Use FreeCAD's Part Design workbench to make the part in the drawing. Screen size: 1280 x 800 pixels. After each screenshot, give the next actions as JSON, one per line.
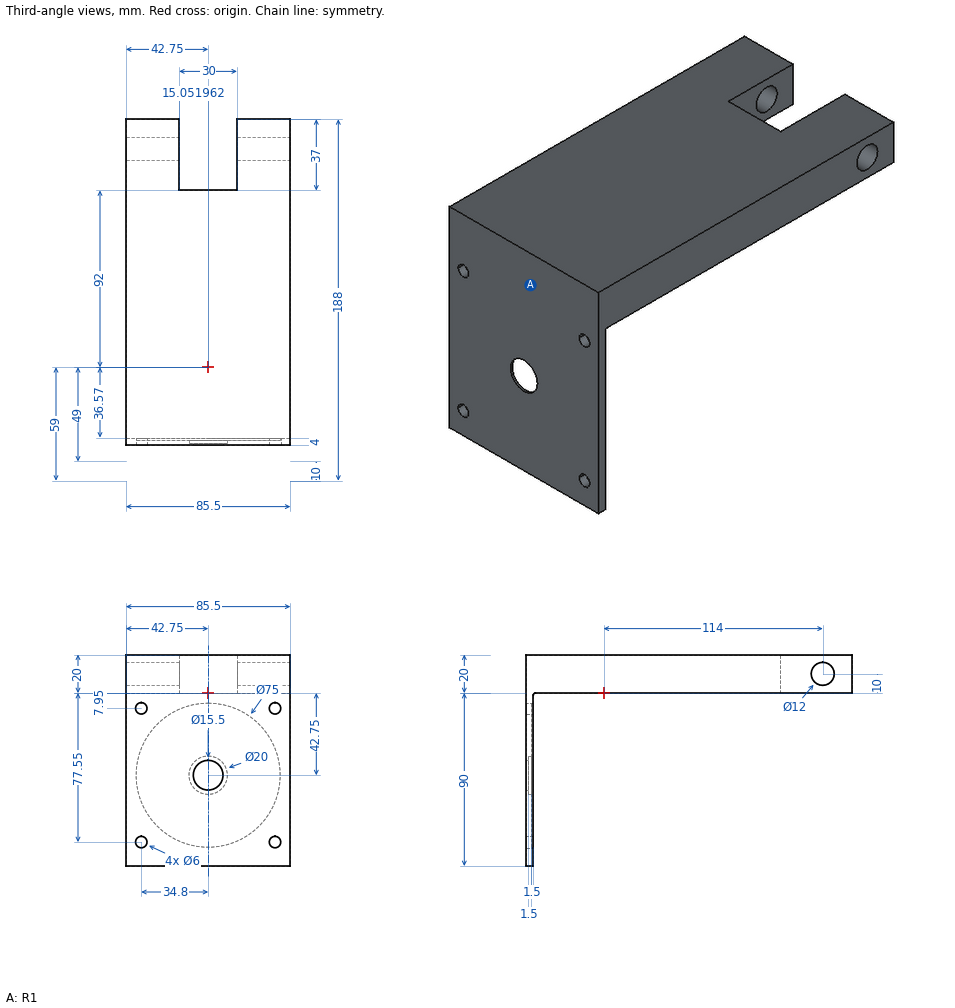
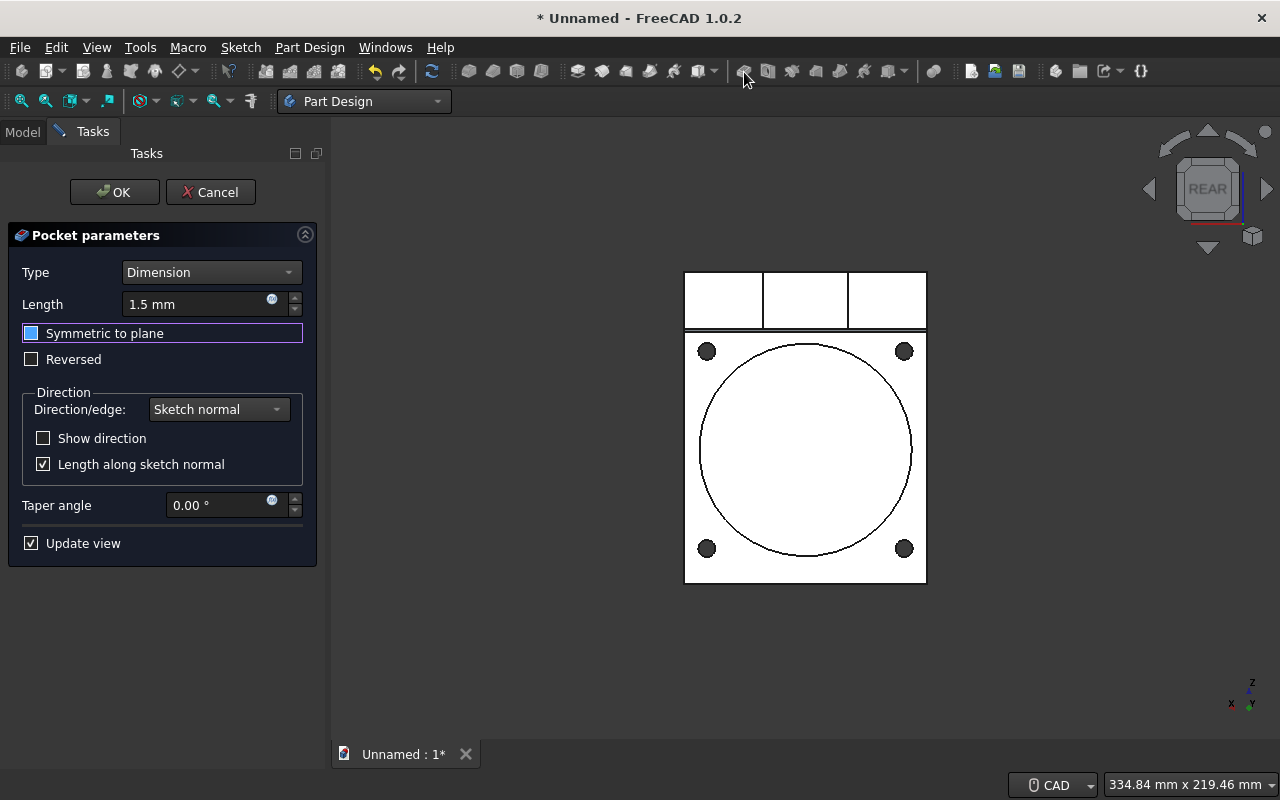
{"action": "left_click", "coordinate": [115, 192]}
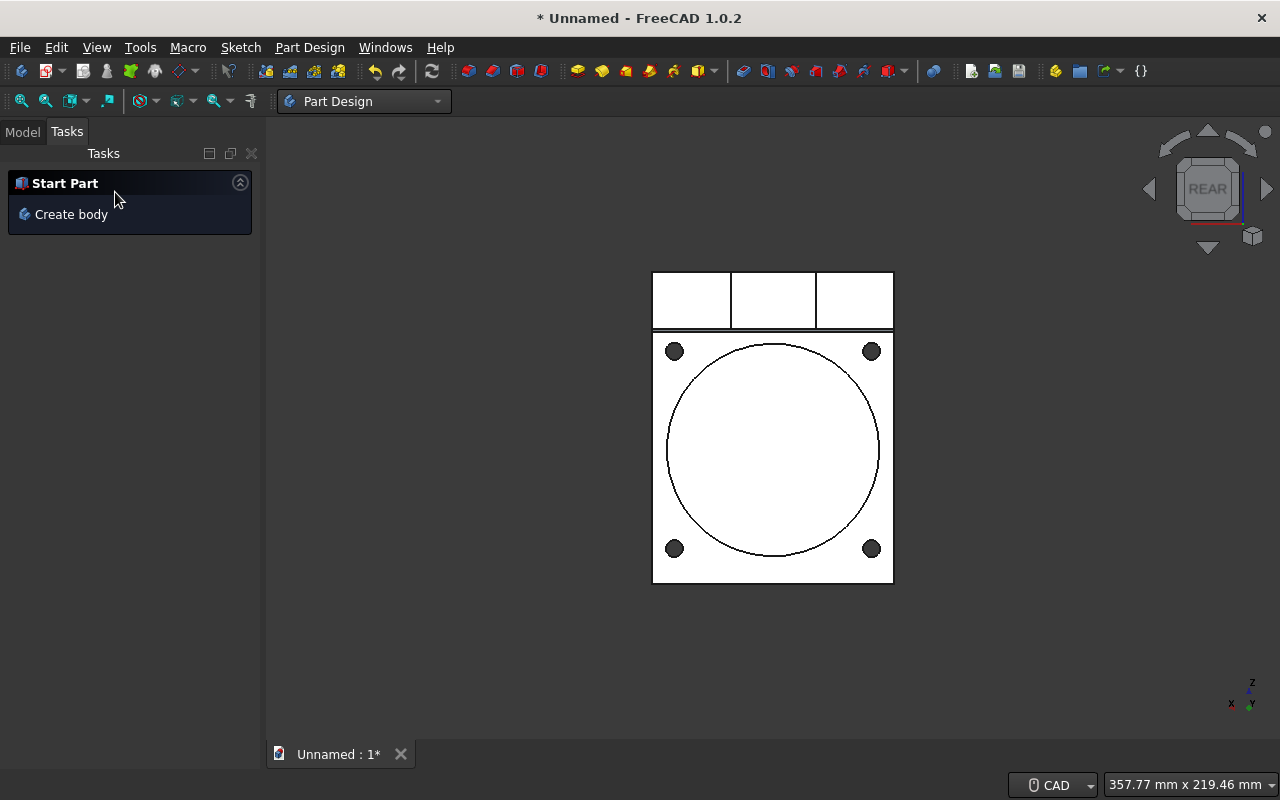
{"action": "left_click", "coordinate": [773, 449]}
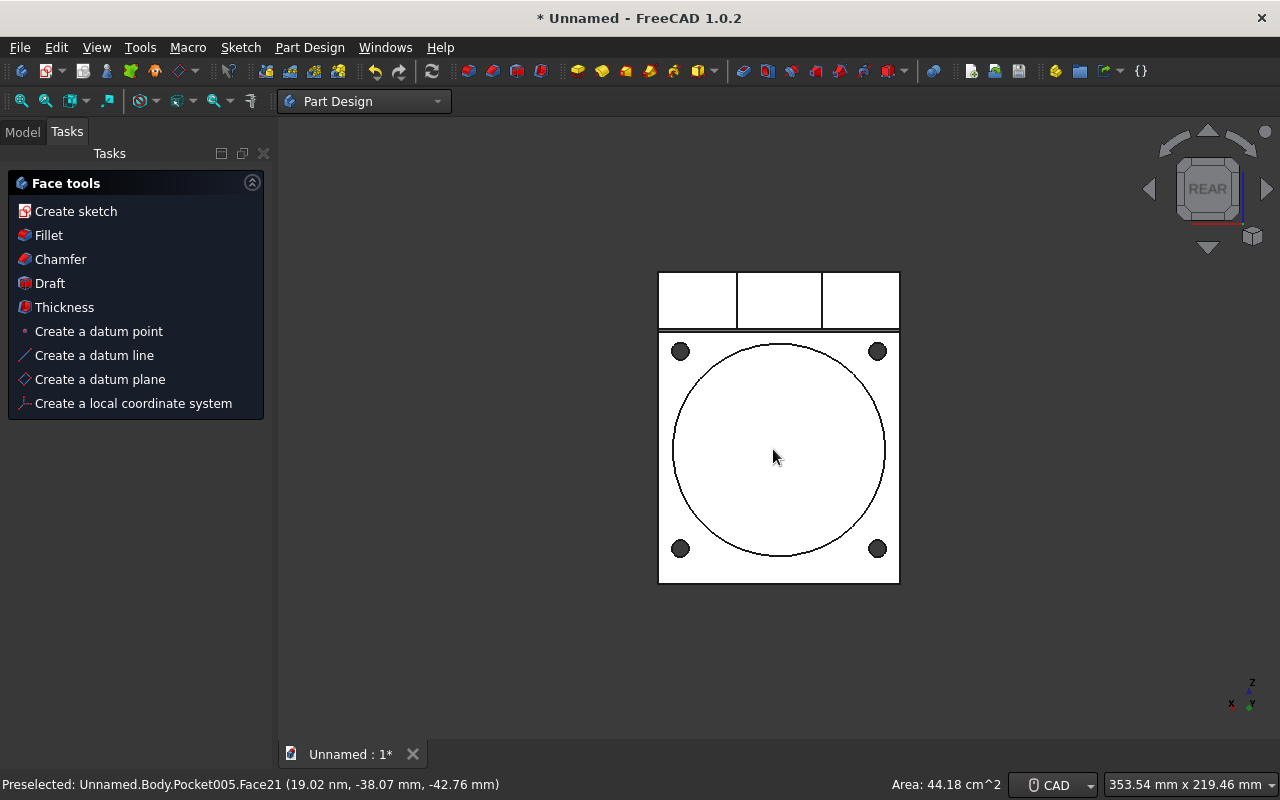
{"action": "left_click", "coordinate": [46, 72]}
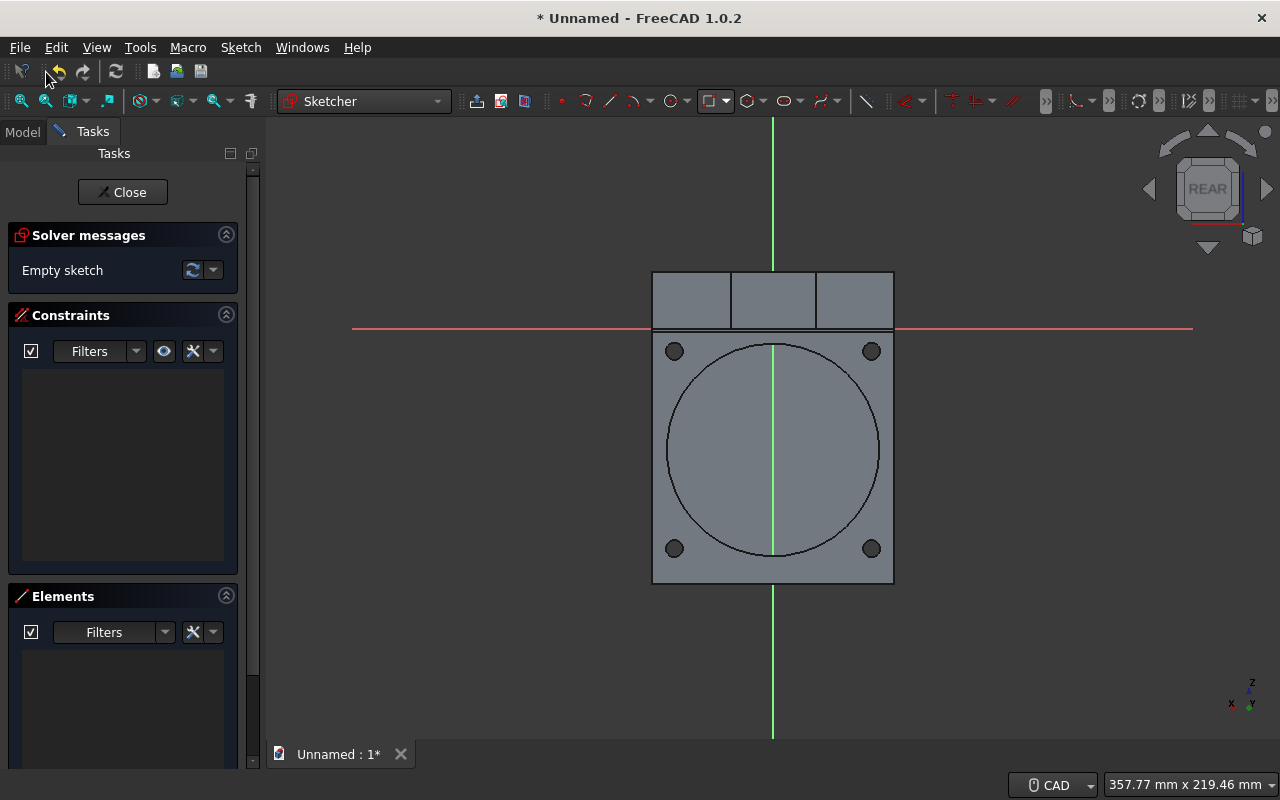
{"action": "key", "text": "q s"}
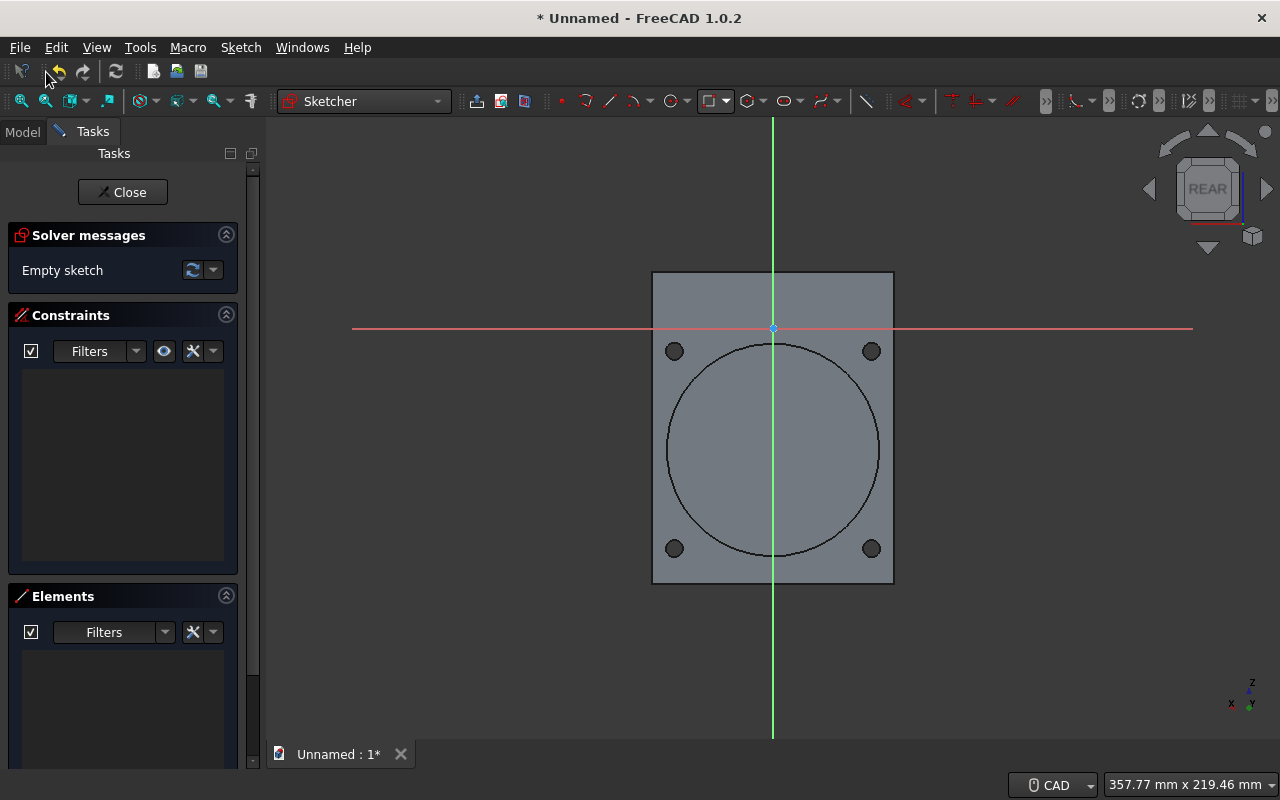
{"action": "scroll", "coordinate": [782, 453], "scroll_direction": "up", "scroll_amount": 11}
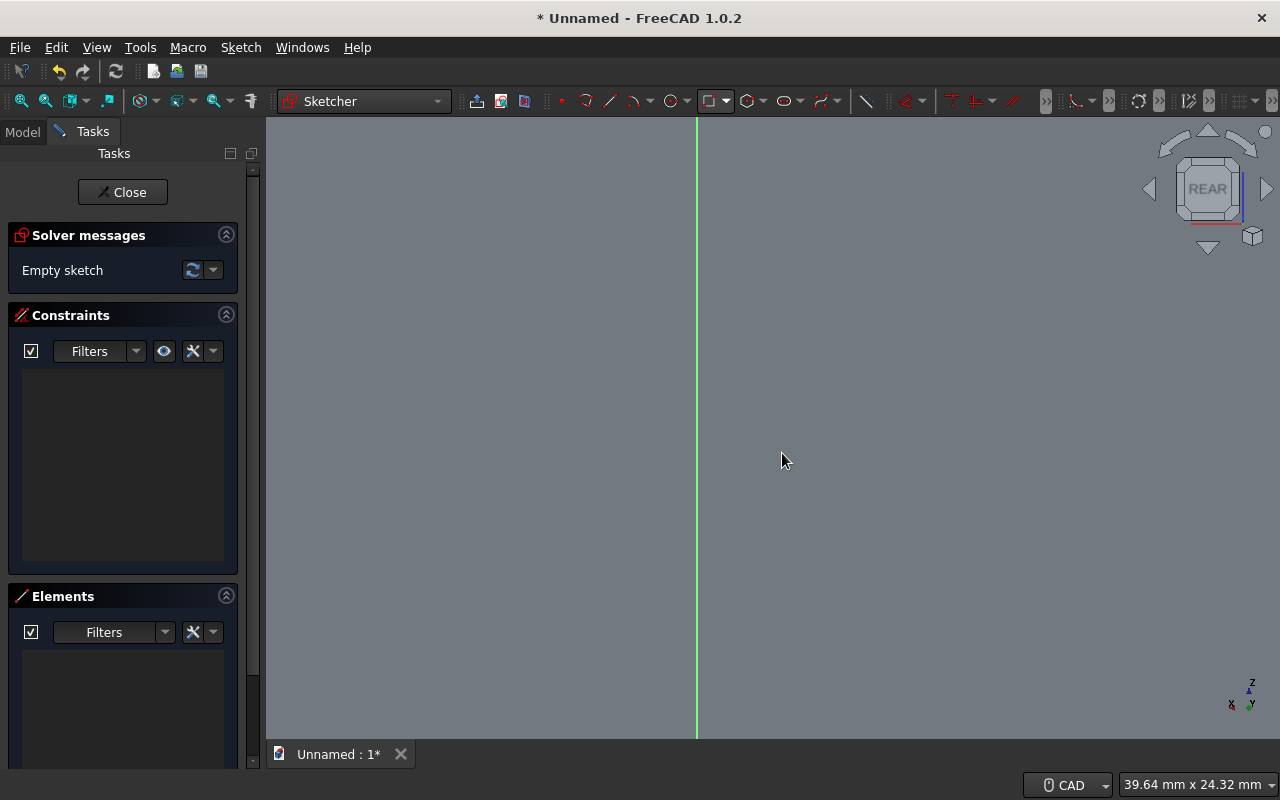
{"action": "left_click", "coordinate": [672, 102]}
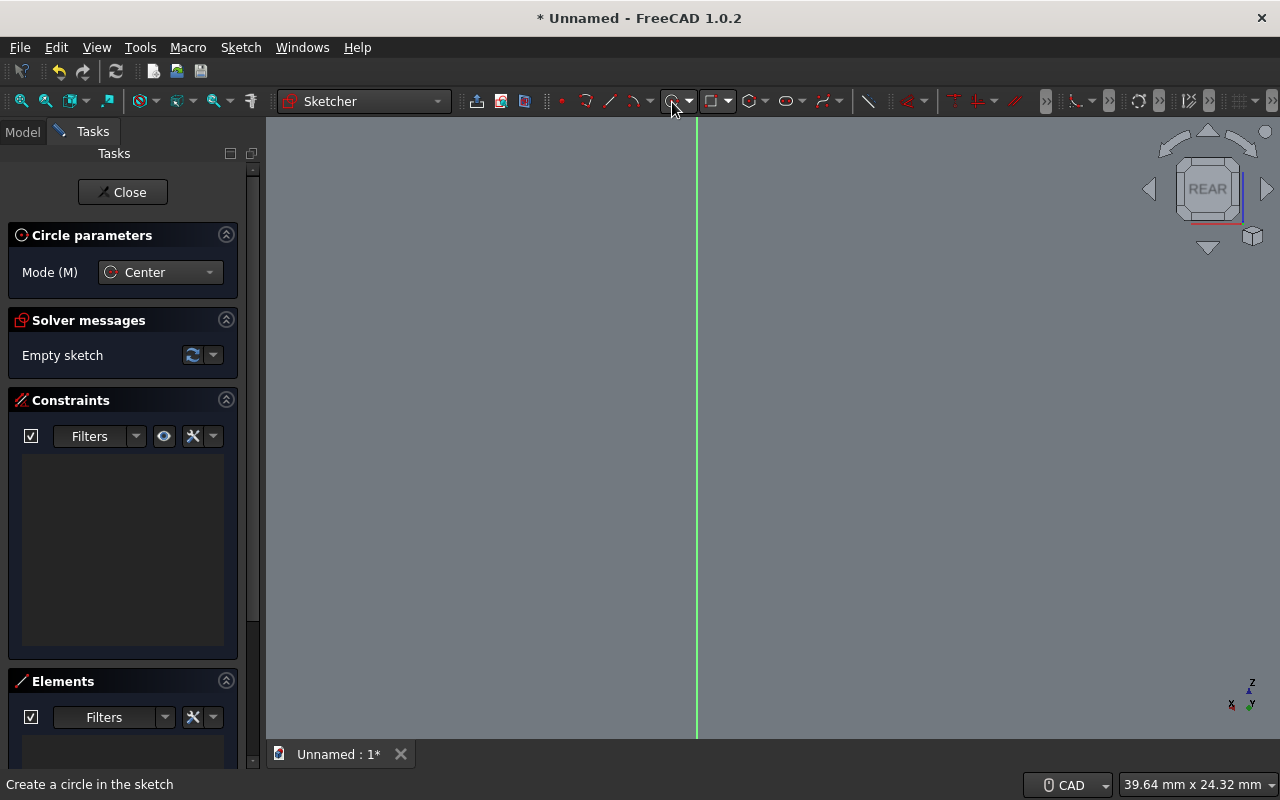
{"action": "left_click", "coordinate": [697, 421]}
{"action": "mouse_move", "coordinate": [837, 281]}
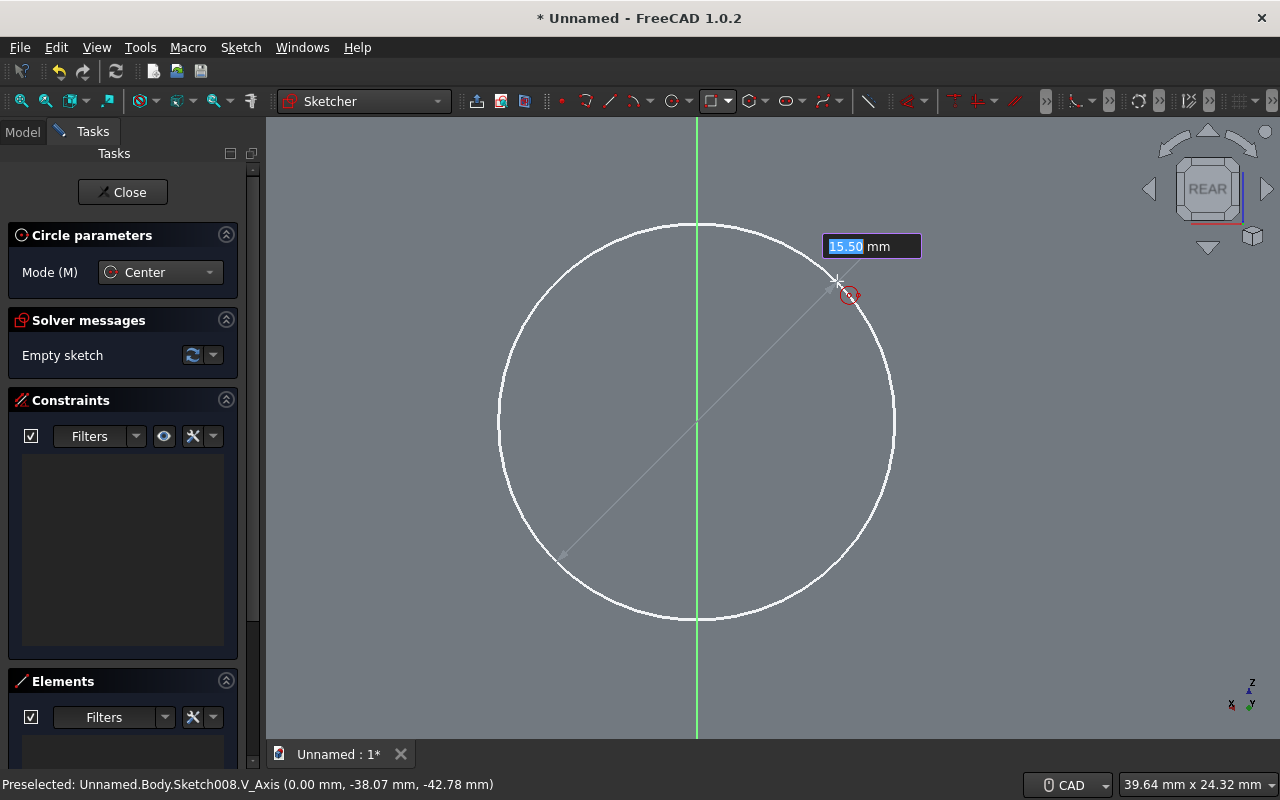
{"action": "type", "text": "15.5"}
{"action": "key", "text": "Return"}
{"action": "key", "text": "Escape"}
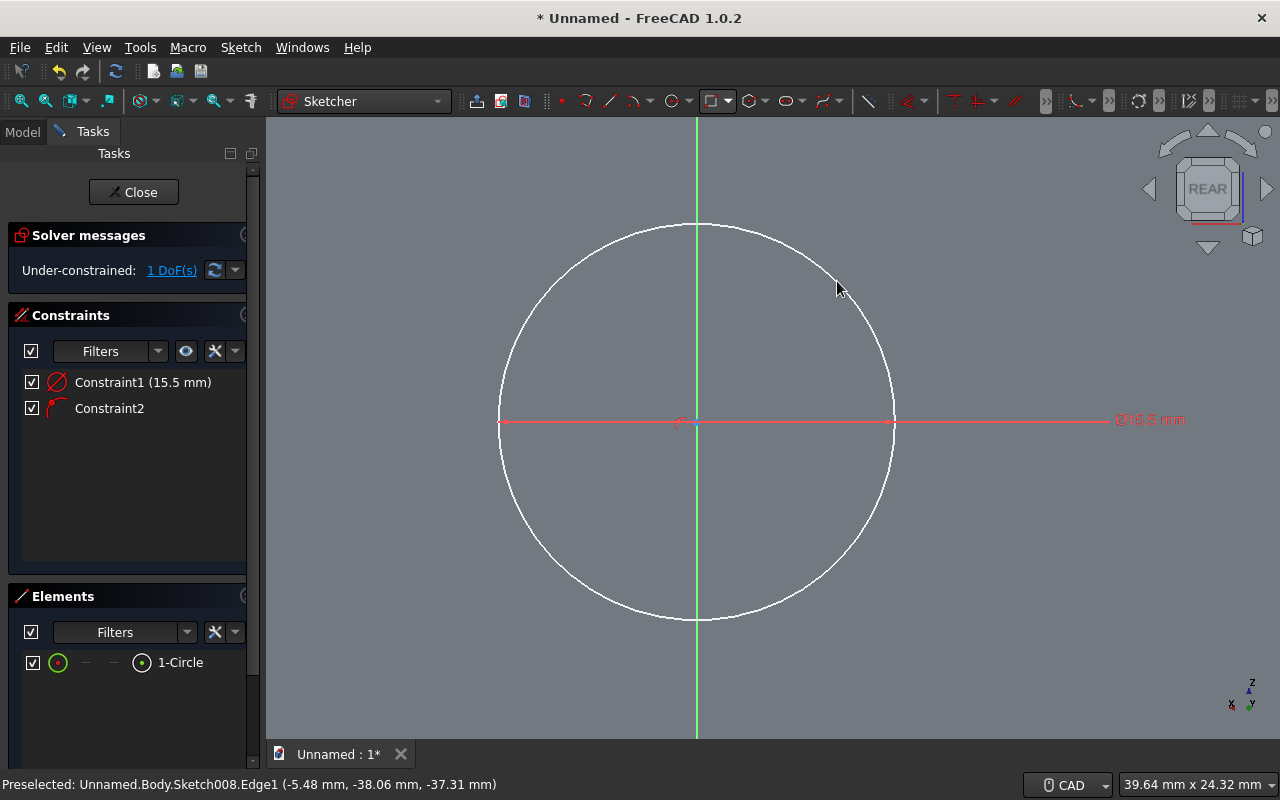
{"action": "key", "text": "d"}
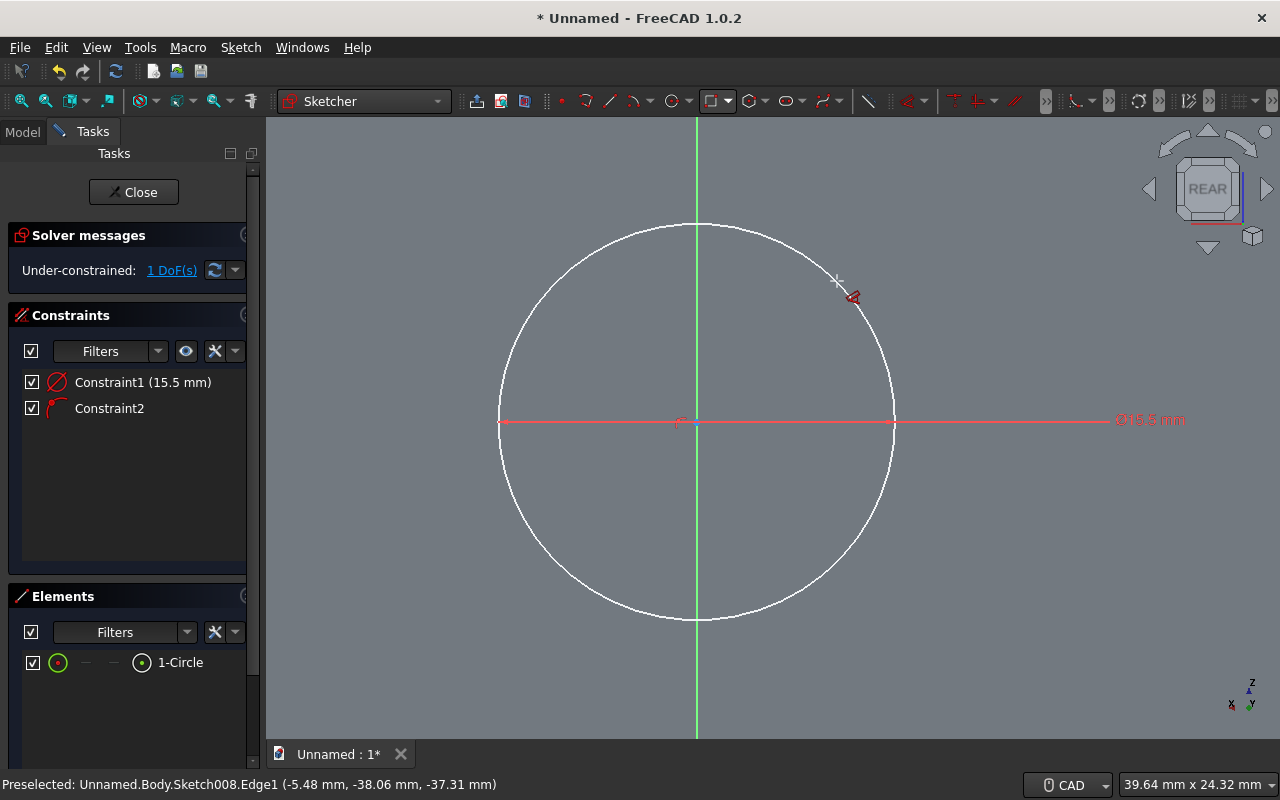
{"action": "left_click", "coordinate": [697, 422]}
{"action": "left_click", "coordinate": [731, 283]}